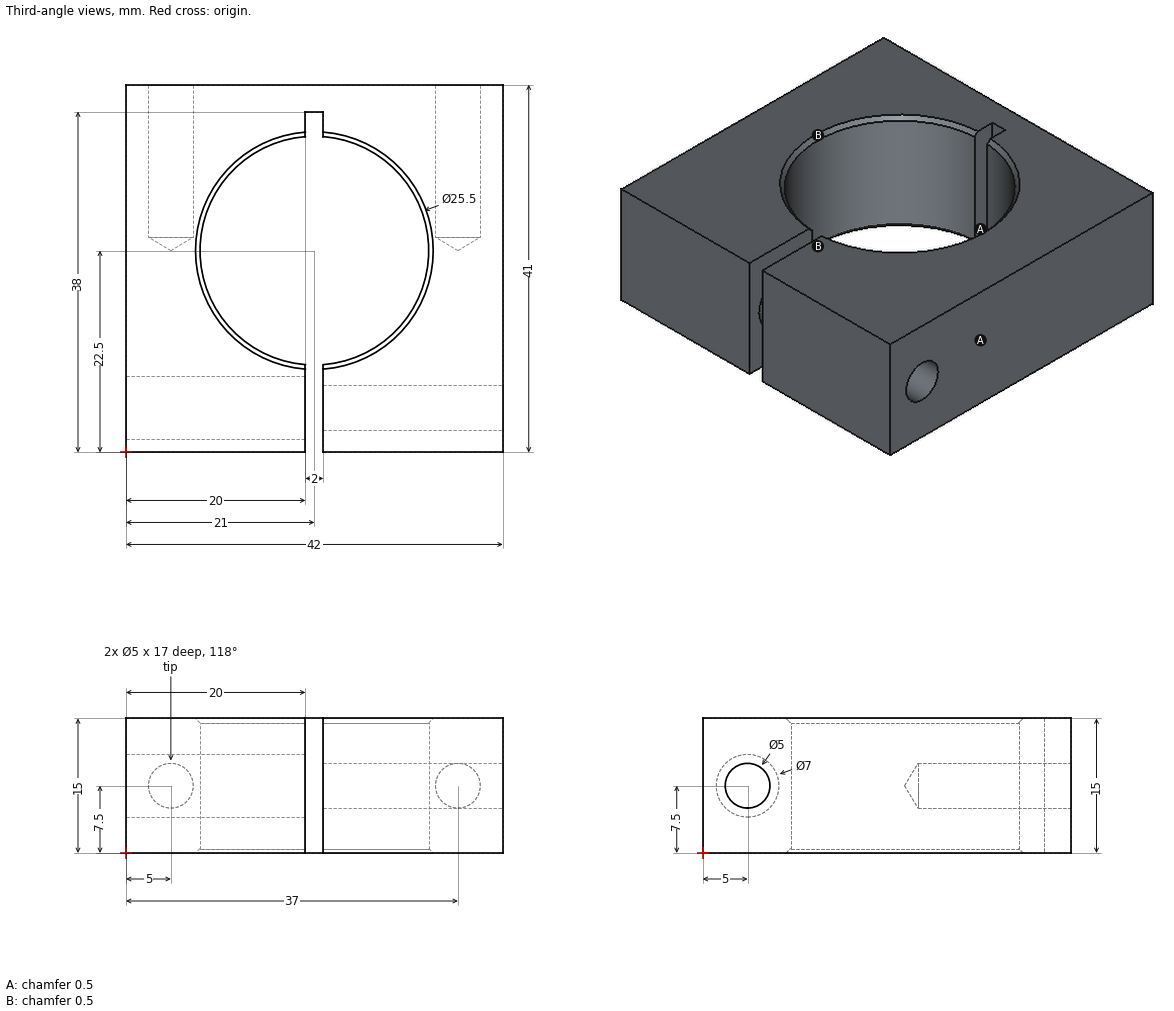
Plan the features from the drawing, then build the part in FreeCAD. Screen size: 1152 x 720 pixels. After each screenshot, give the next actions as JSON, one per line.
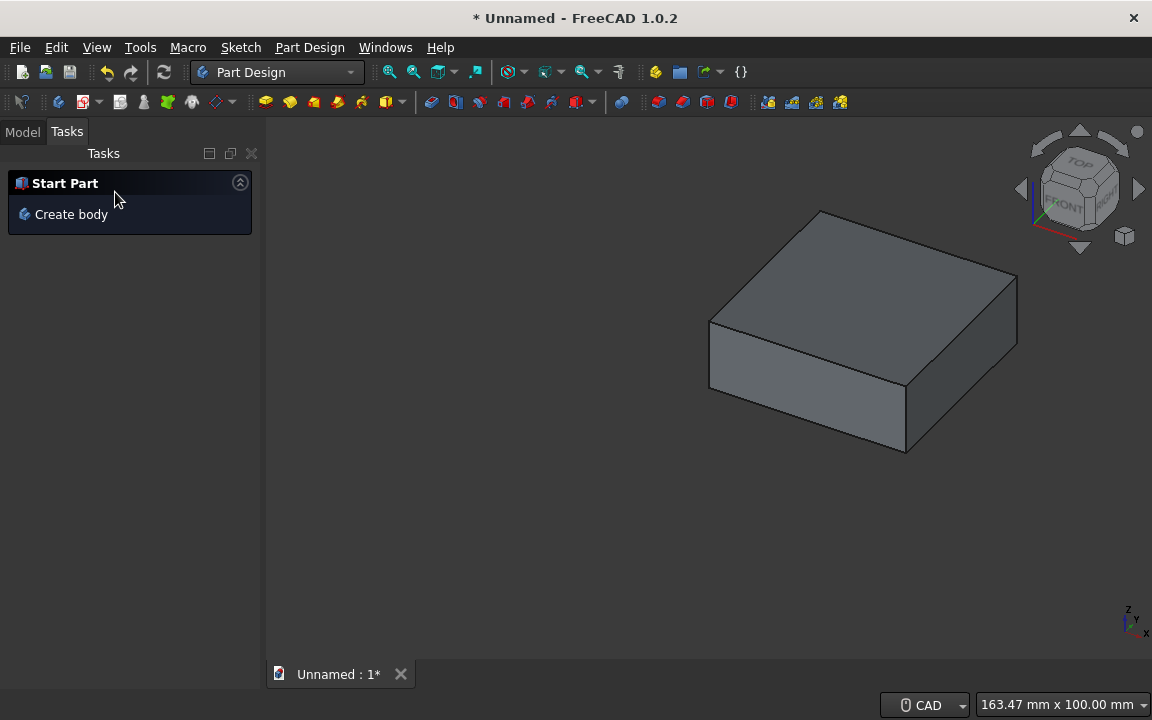
{"action": "left_click", "coordinate": [390, 72]}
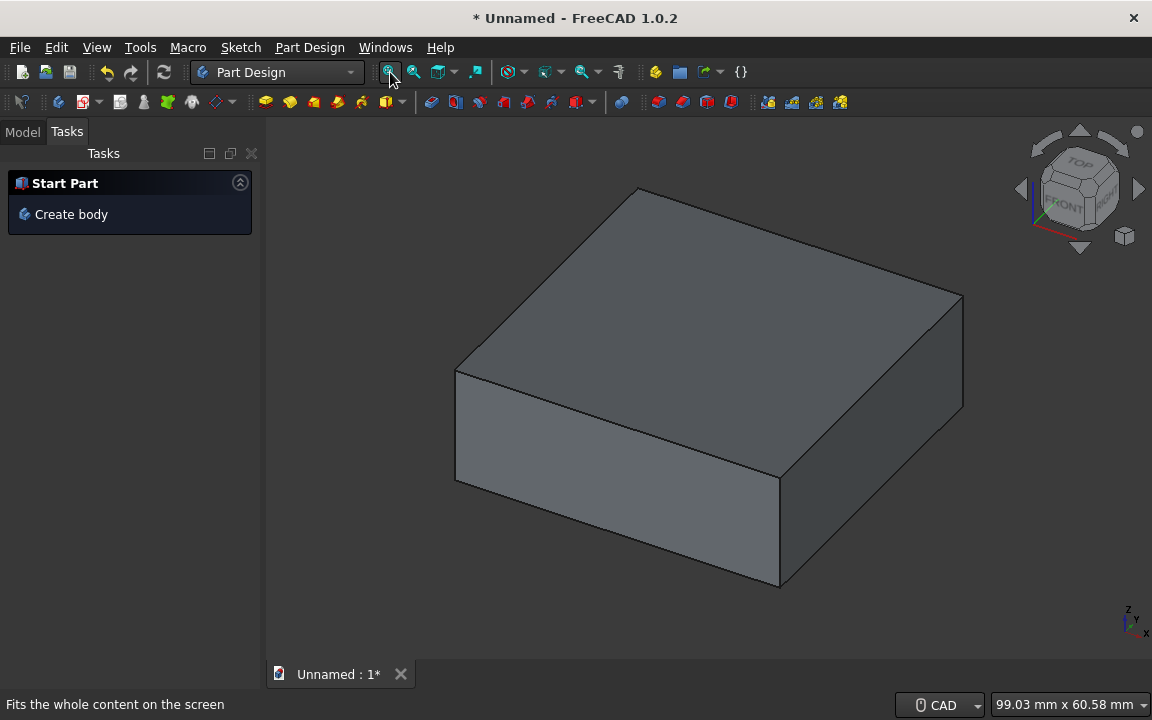
{"action": "left_click", "coordinate": [709, 332]}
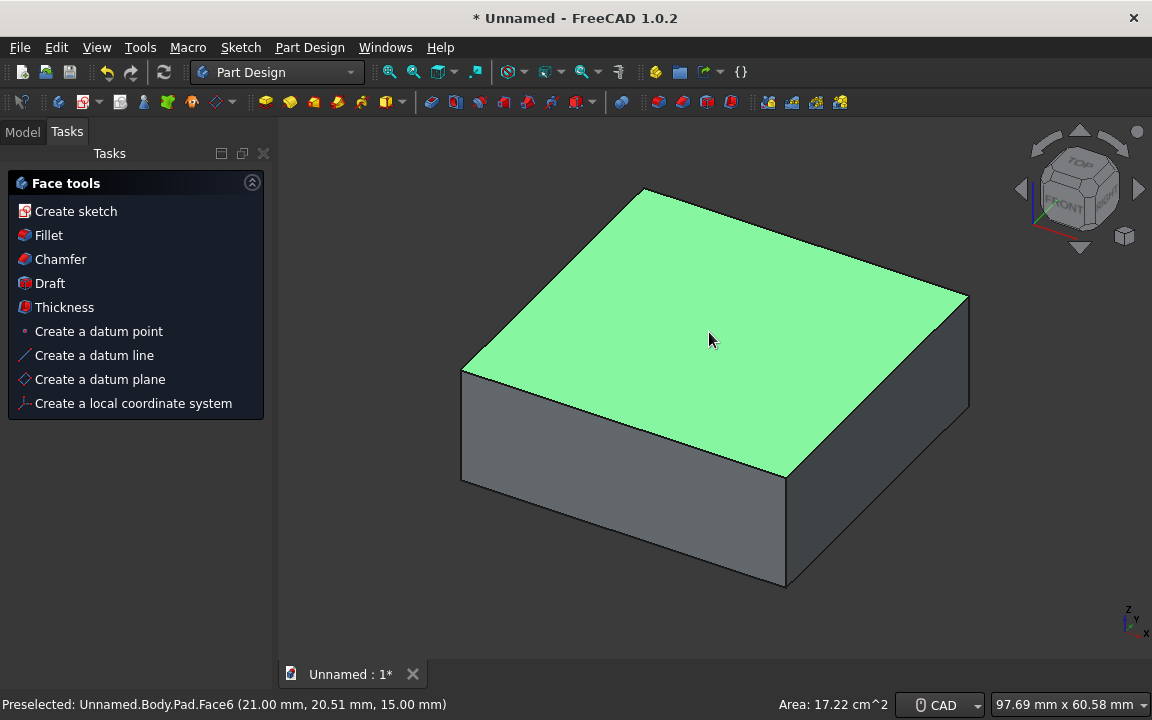
{"action": "left_click", "coordinate": [84, 102]}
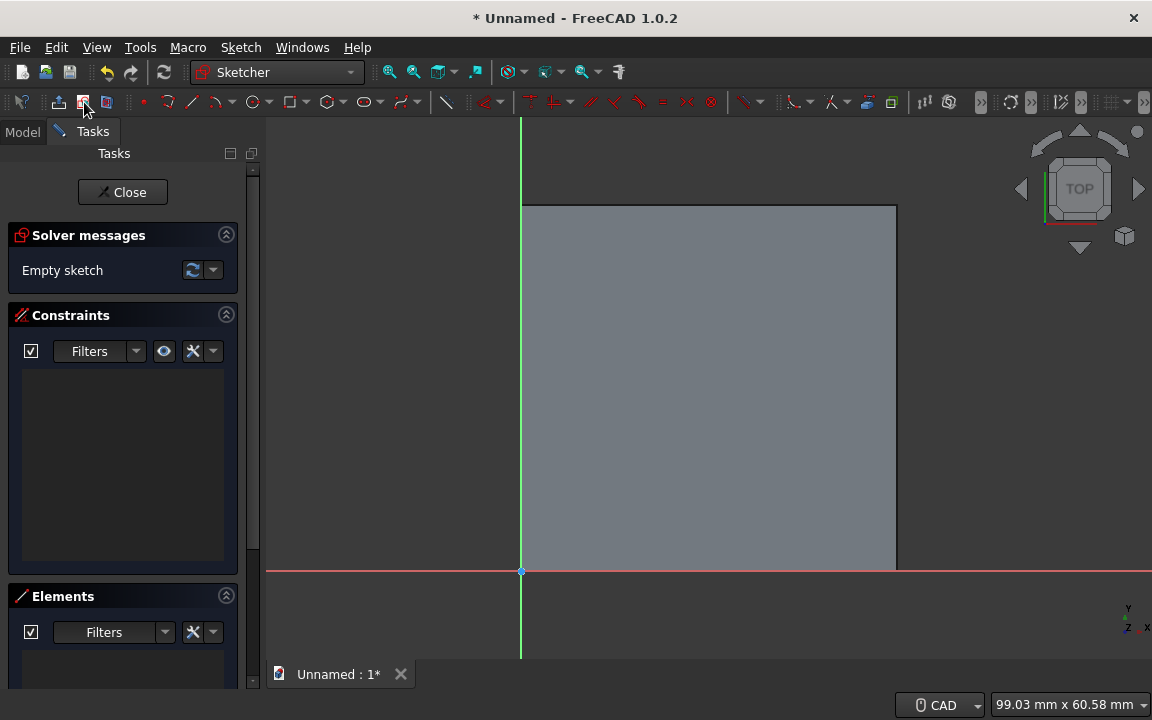
{"action": "left_click", "coordinate": [254, 102]}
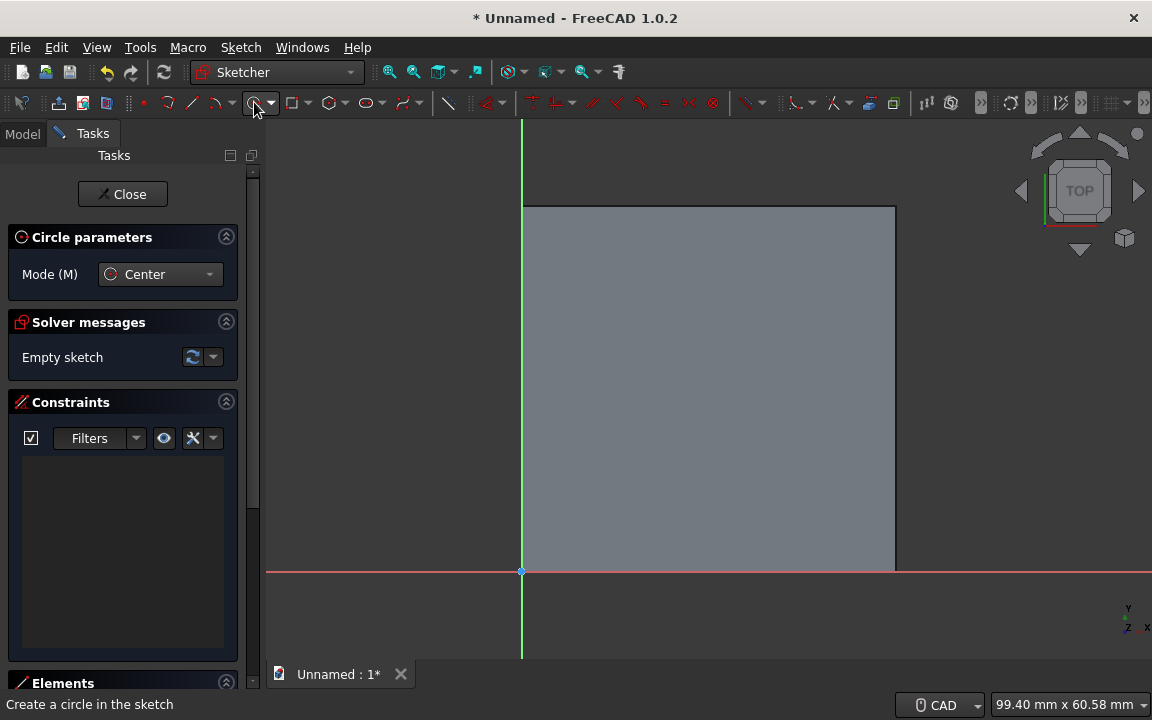
{"action": "left_click", "coordinate": [709, 371]}
{"action": "mouse_move", "coordinate": [789, 291]}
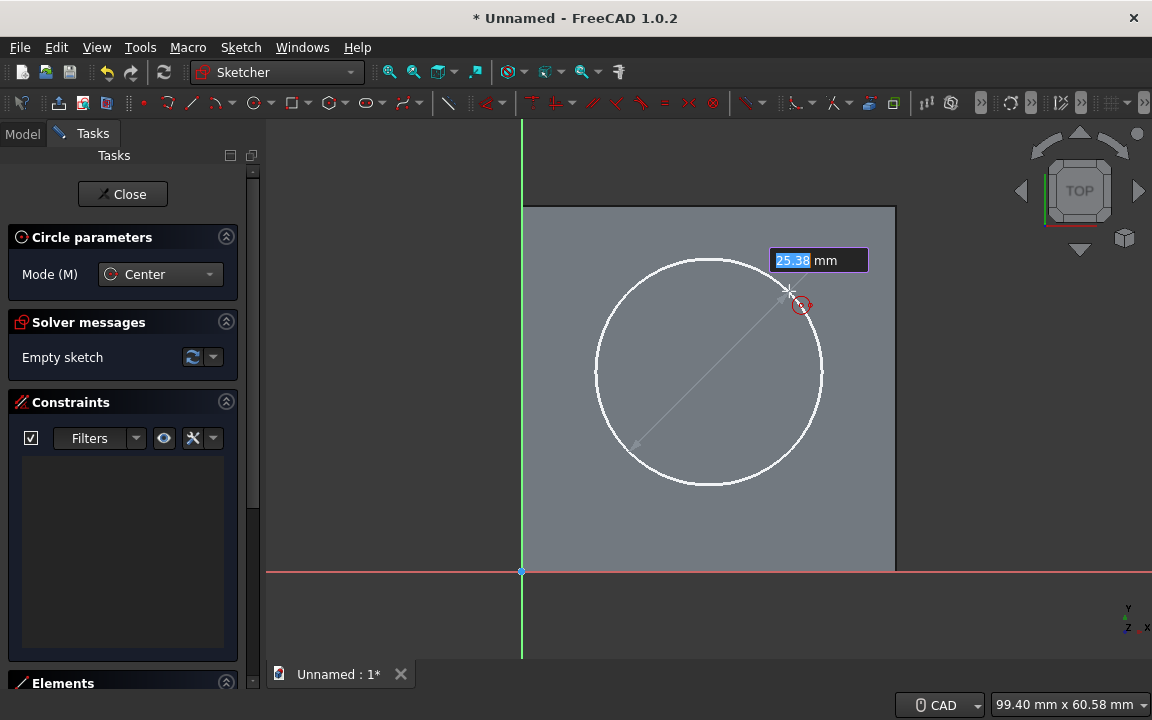
{"action": "type", "text": "25.5"}
{"action": "key", "text": "Return"}
{"action": "key", "text": "Escape"}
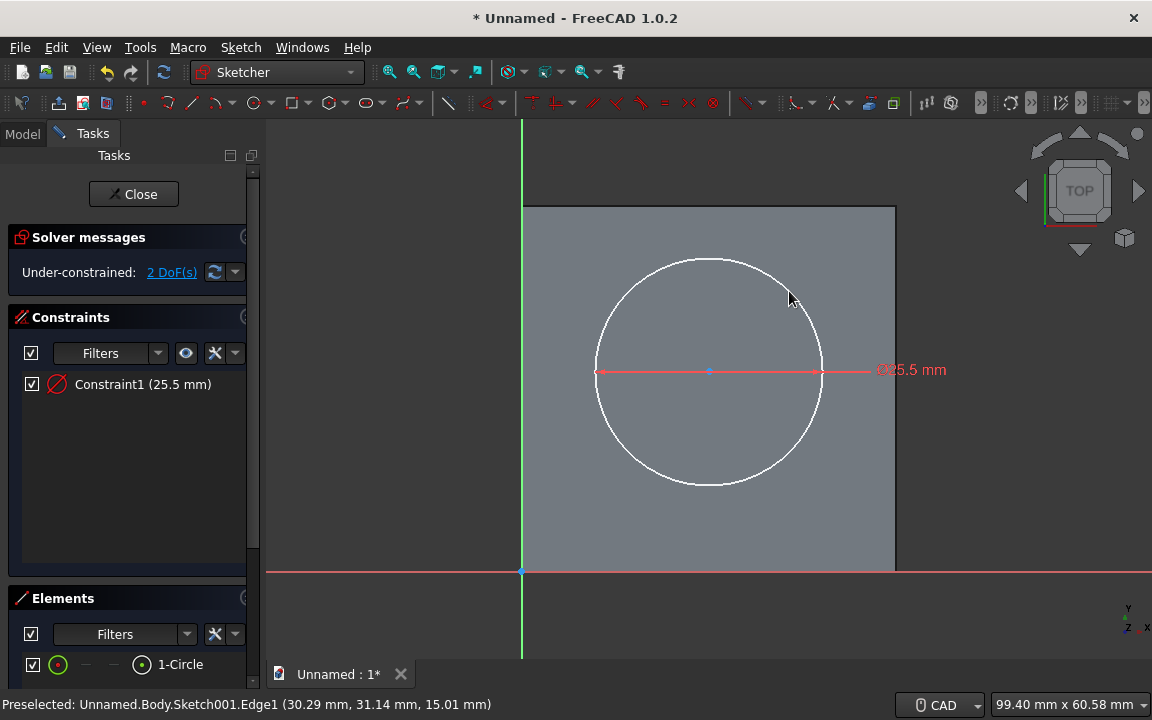
{"action": "left_click", "coordinate": [709, 372]}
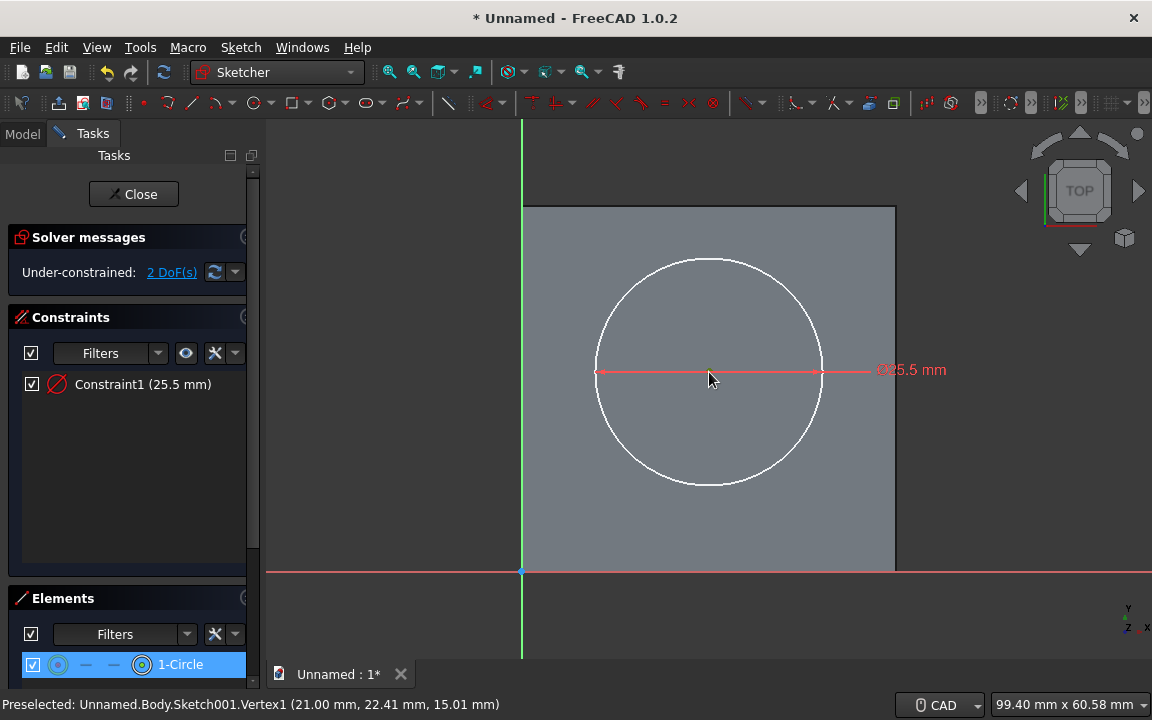
{"action": "left_click", "coordinate": [504, 104]}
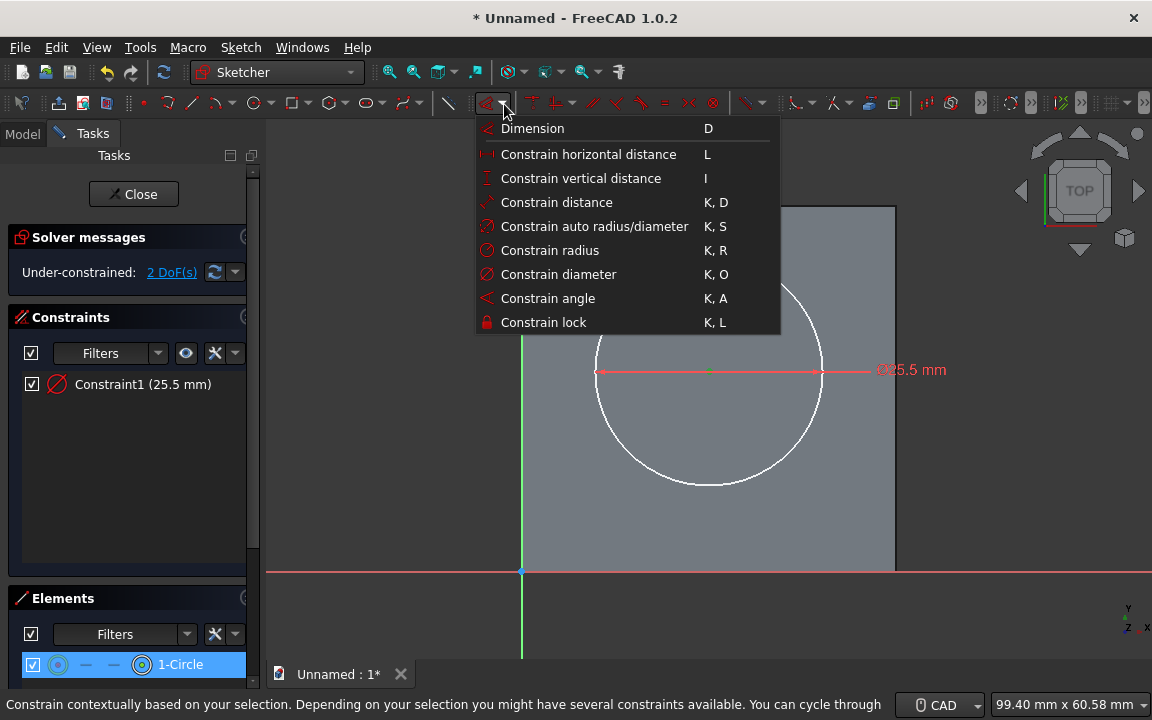
{"action": "left_click", "coordinate": [628, 154]}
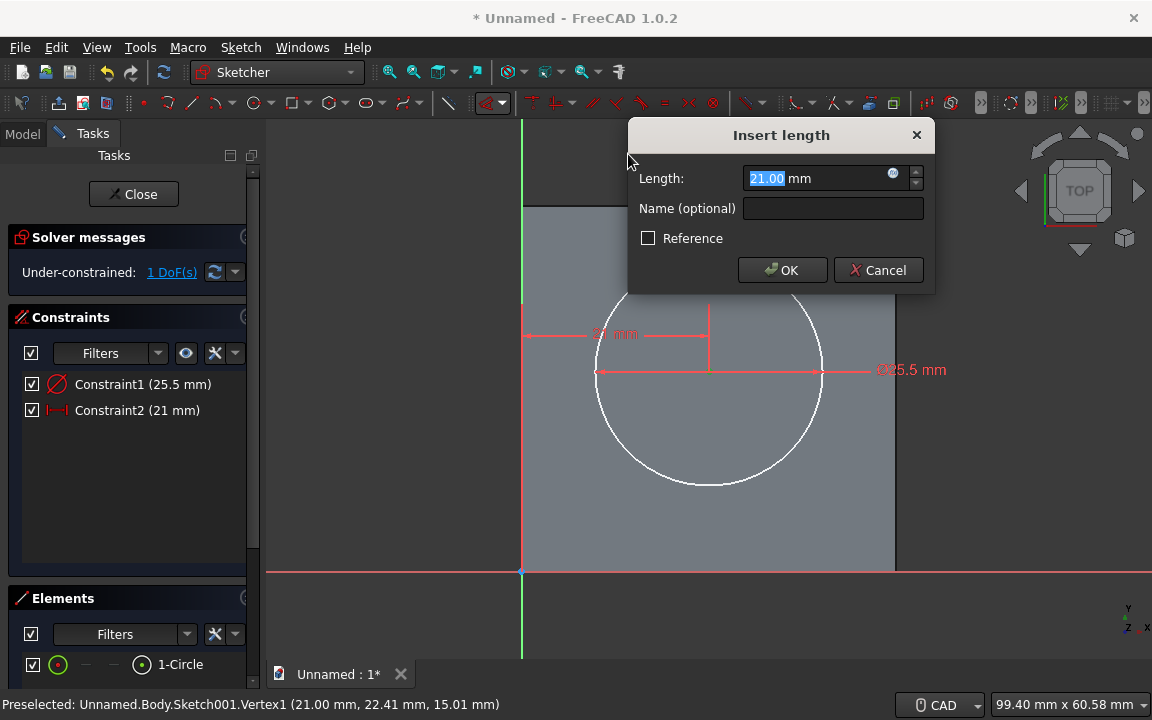
{"action": "type", "text": "21"}
{"action": "key", "text": "Return"}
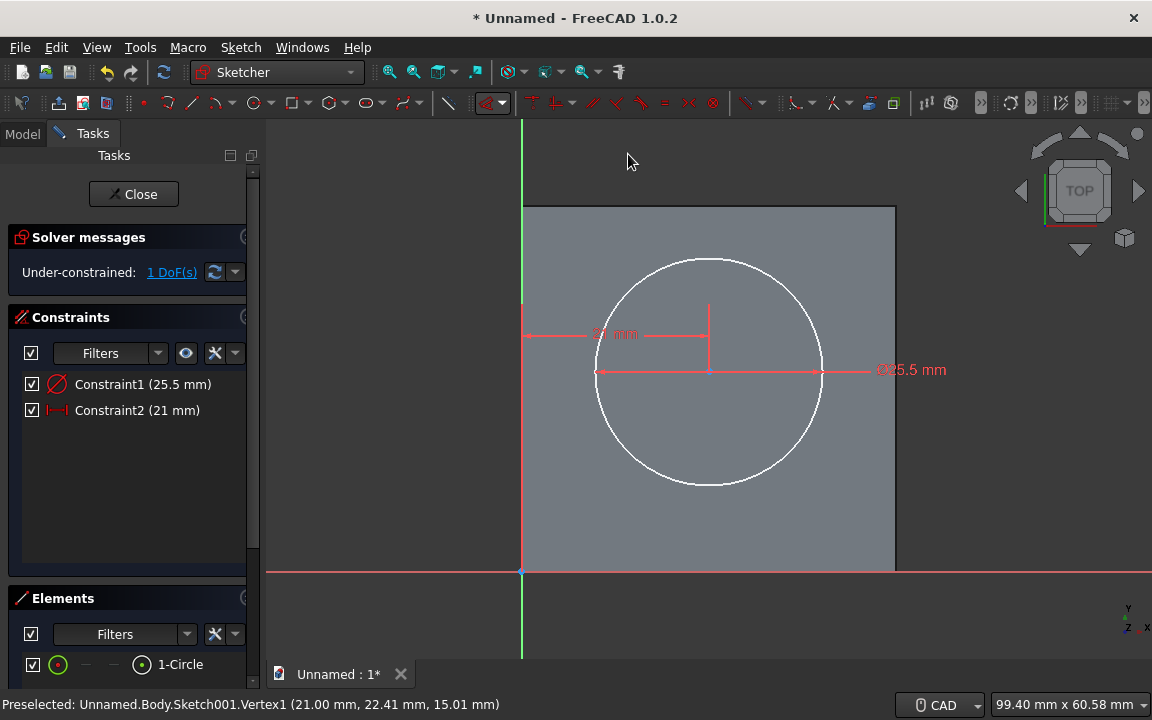
{"action": "left_click", "coordinate": [709, 372]}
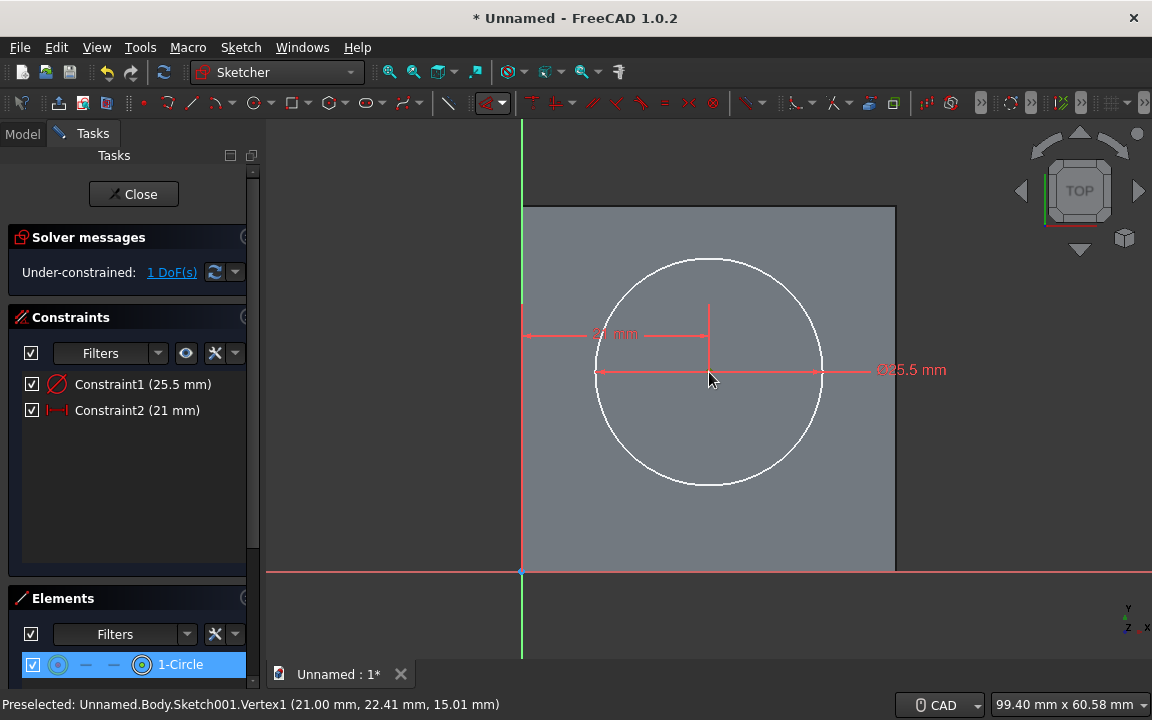
{"action": "left_click", "coordinate": [504, 104]}